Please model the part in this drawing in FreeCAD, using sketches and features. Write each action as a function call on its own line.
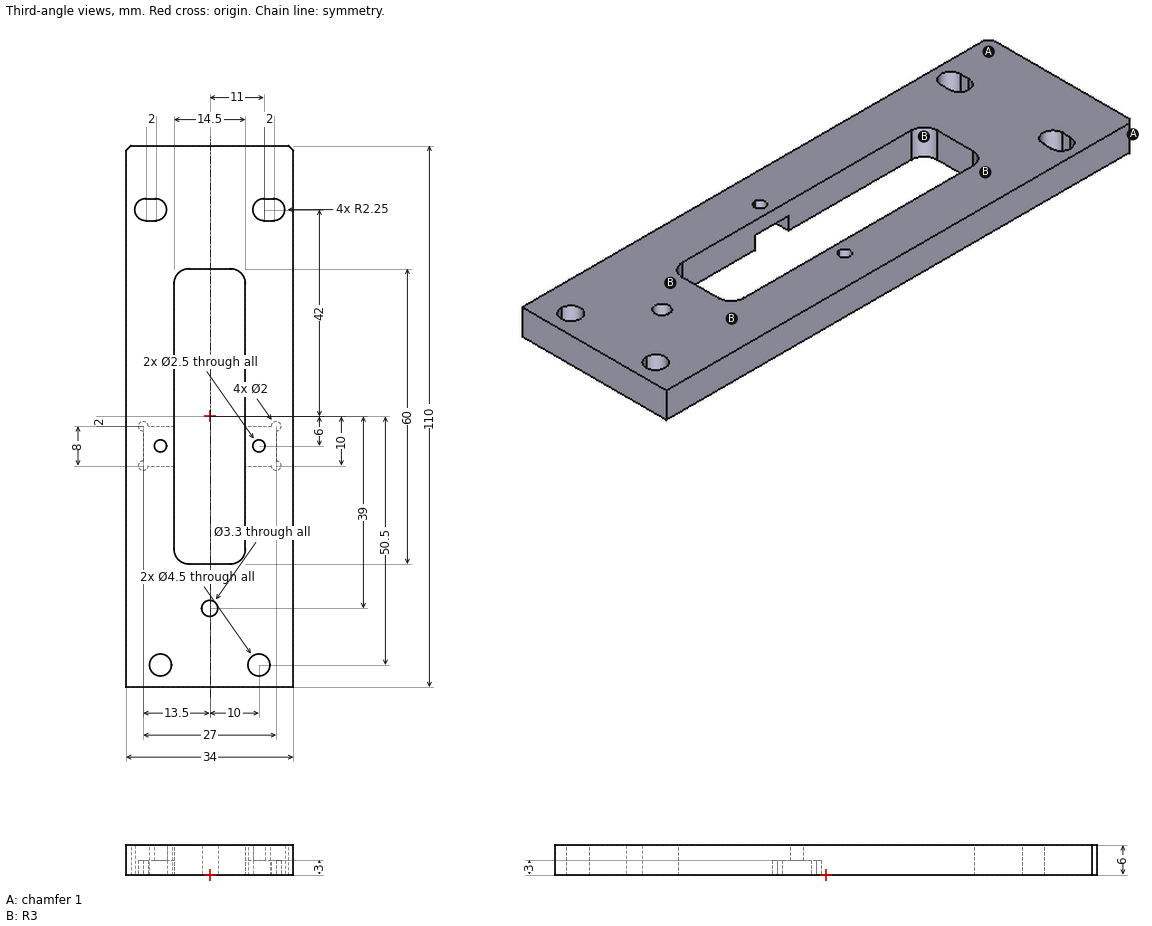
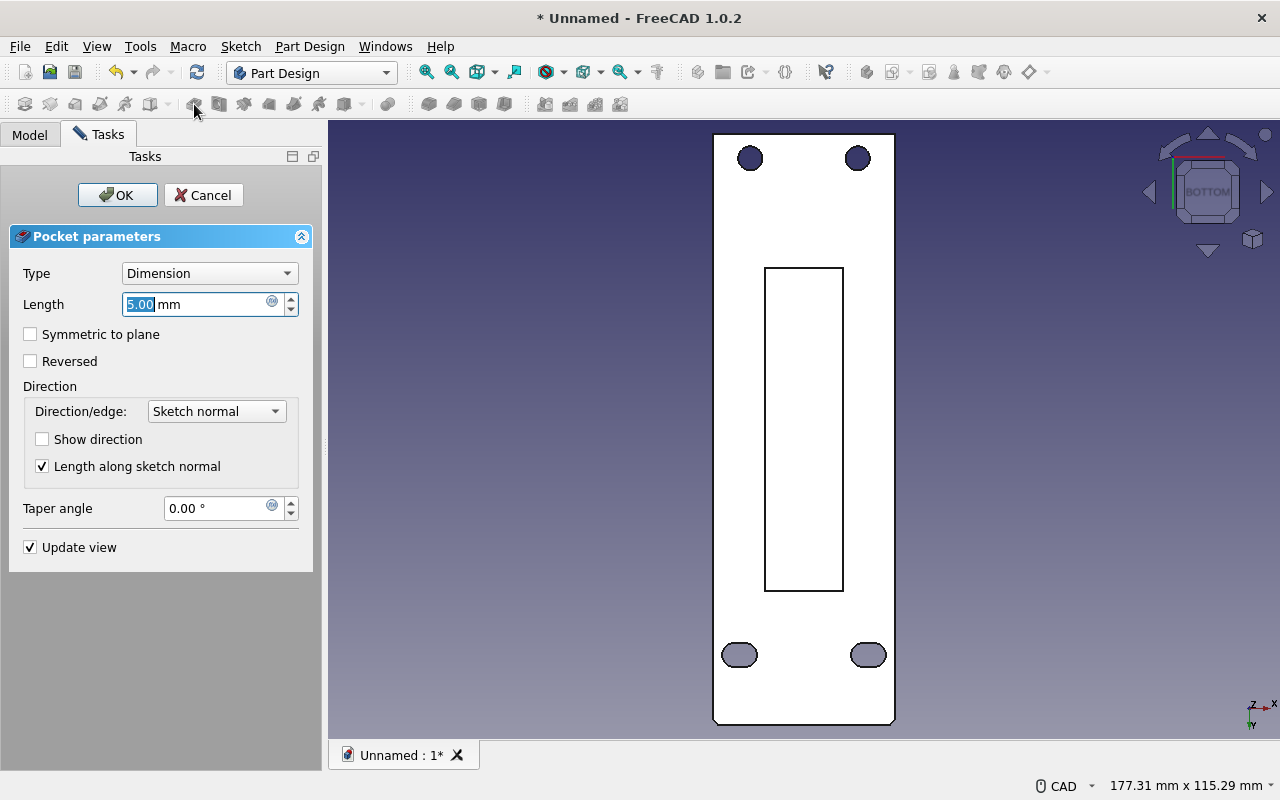
click(210, 274)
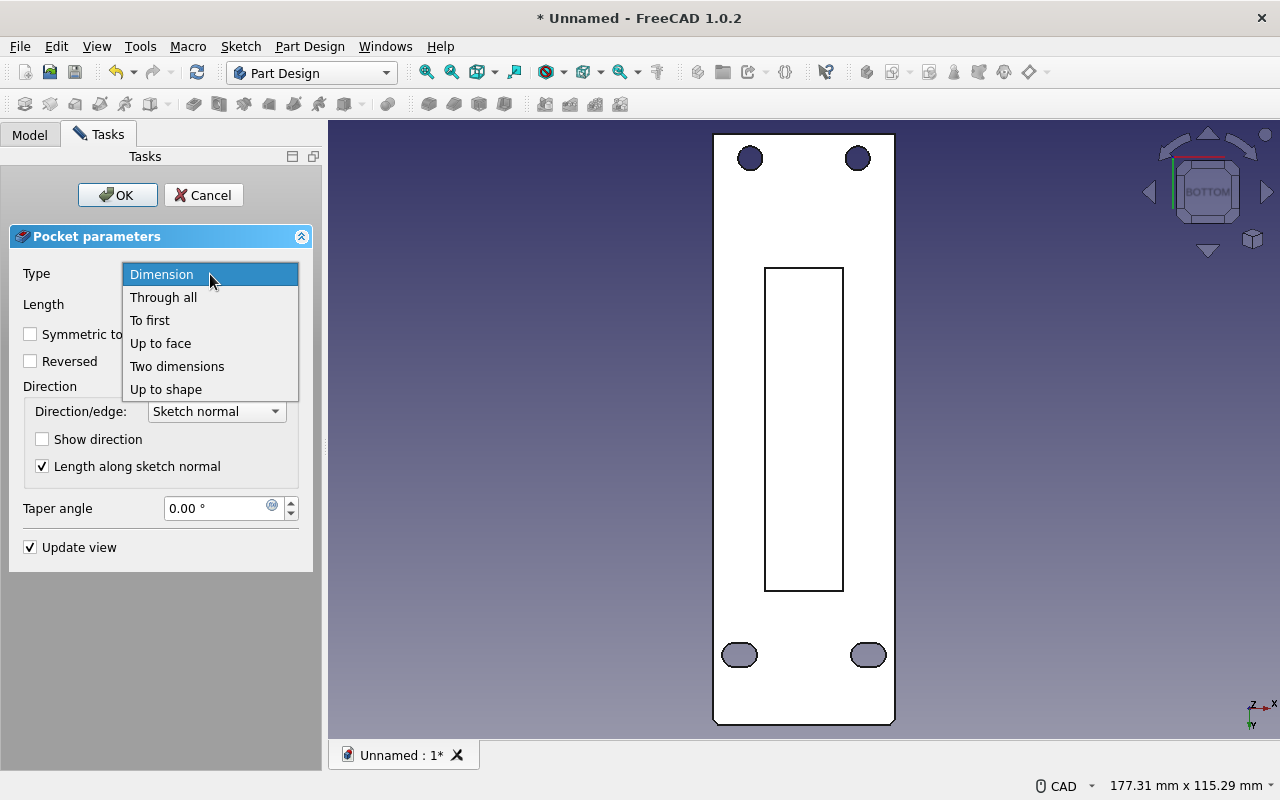
click(208, 298)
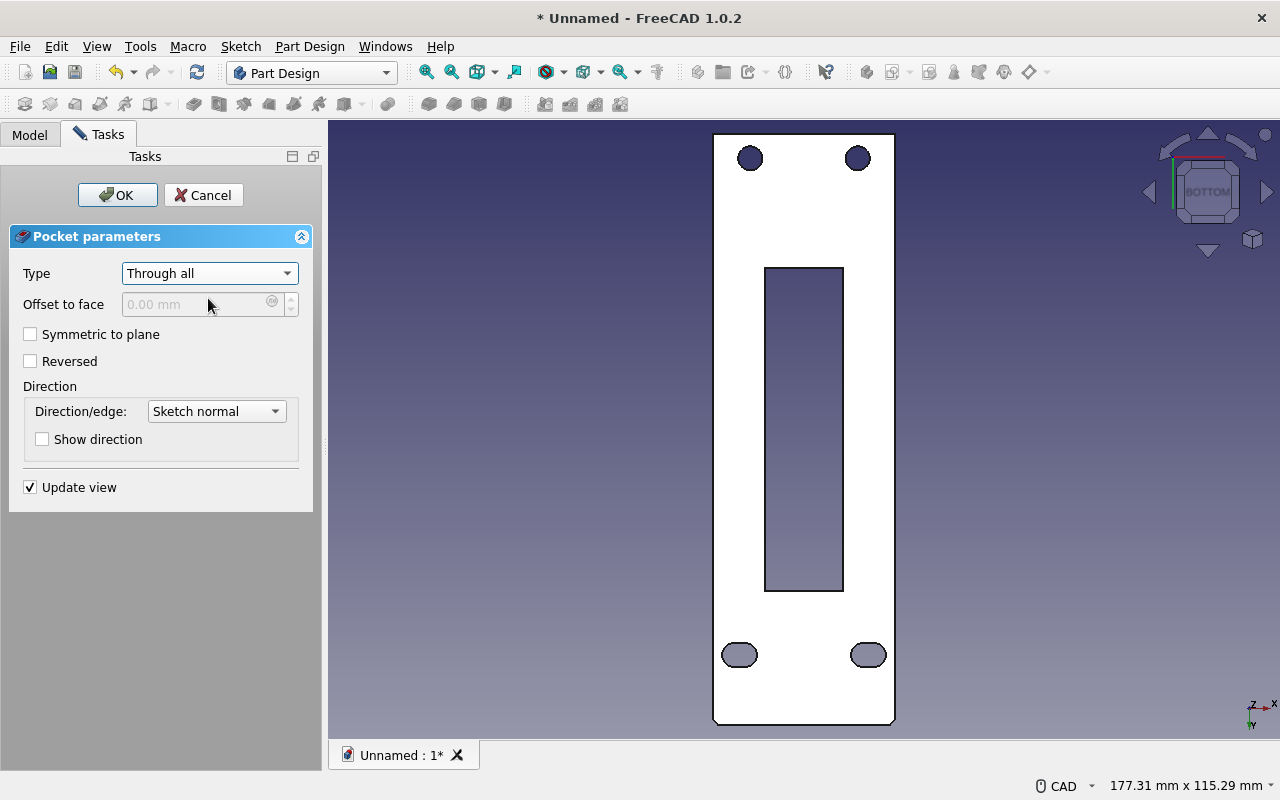
click(118, 195)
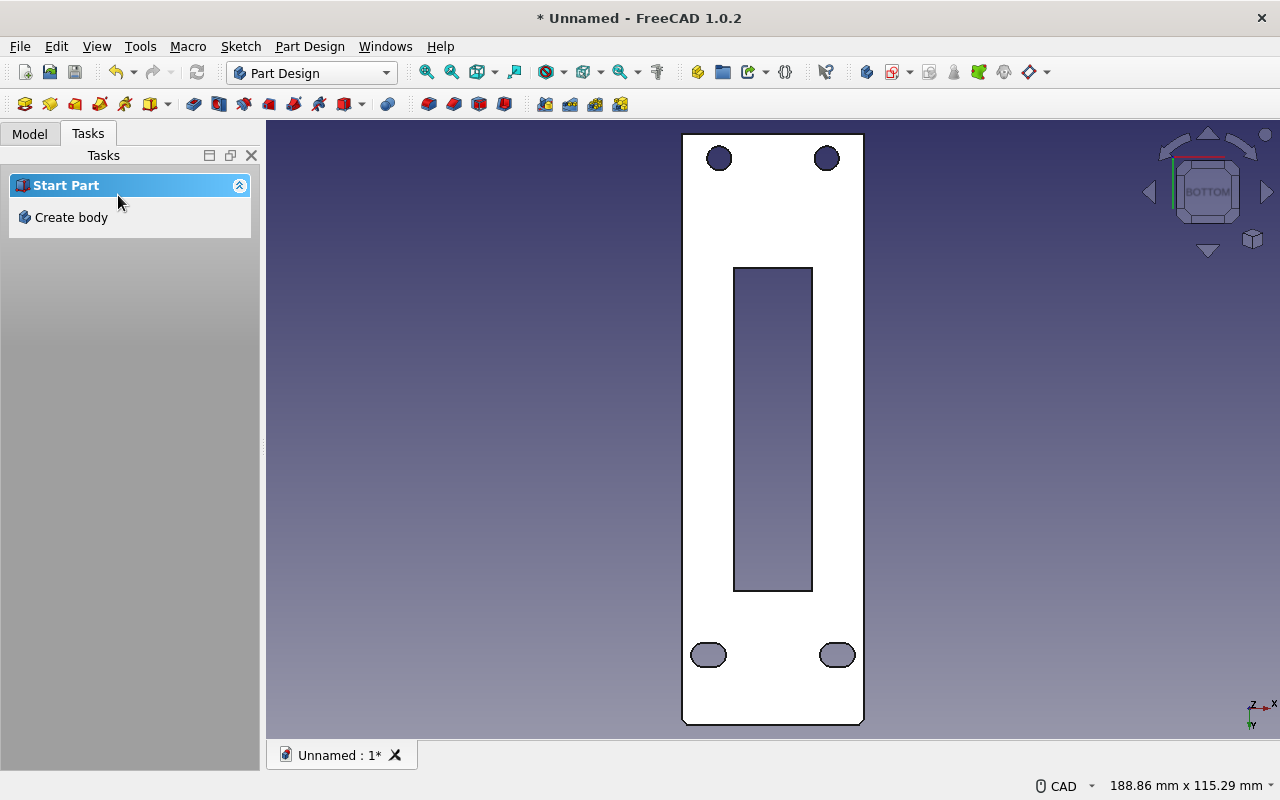
click(773, 682)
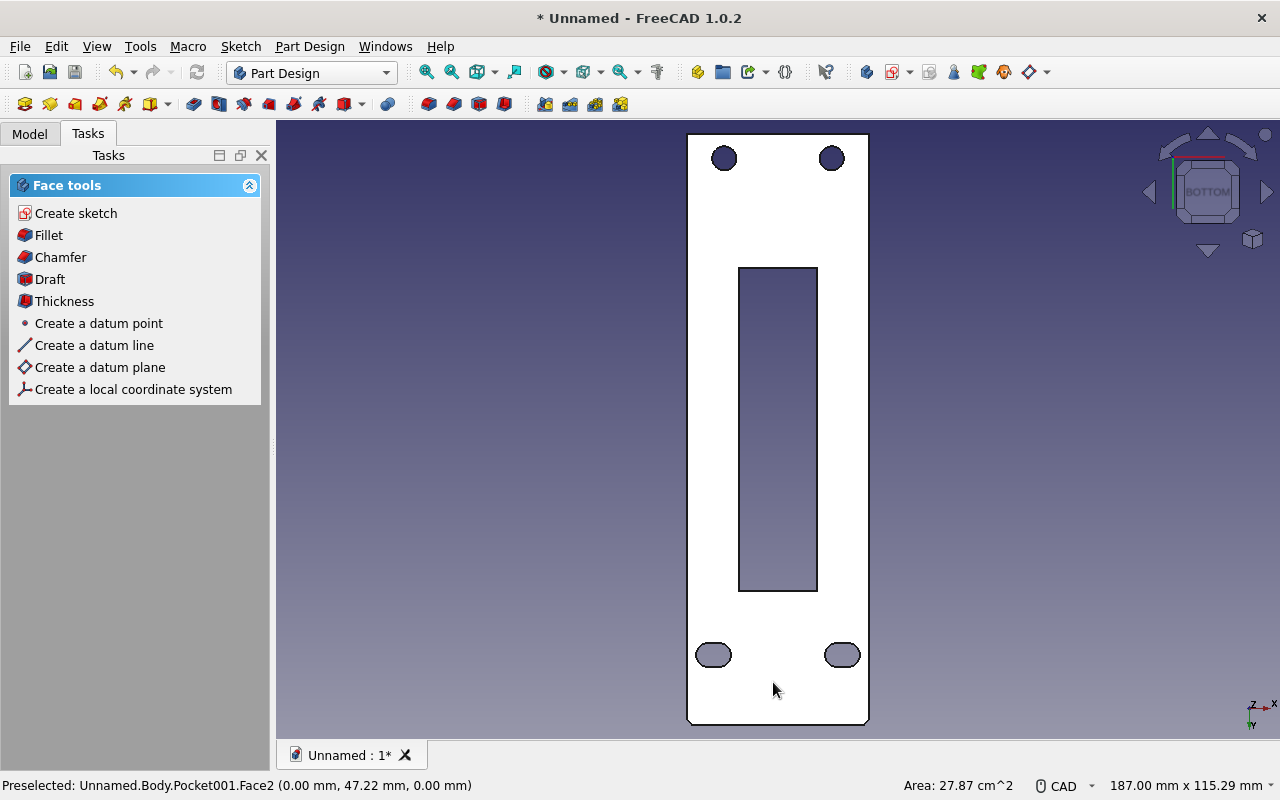
click(892, 72)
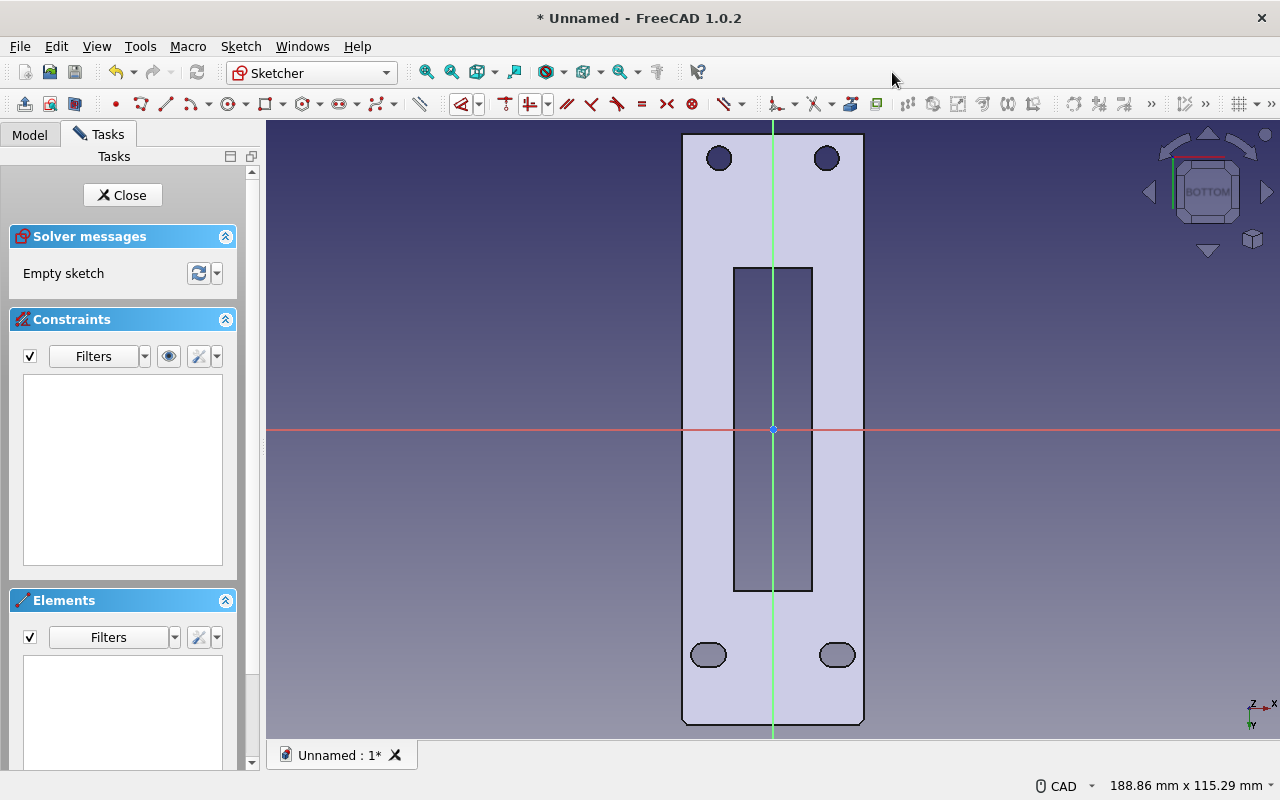
scroll(795, 394, up, 7)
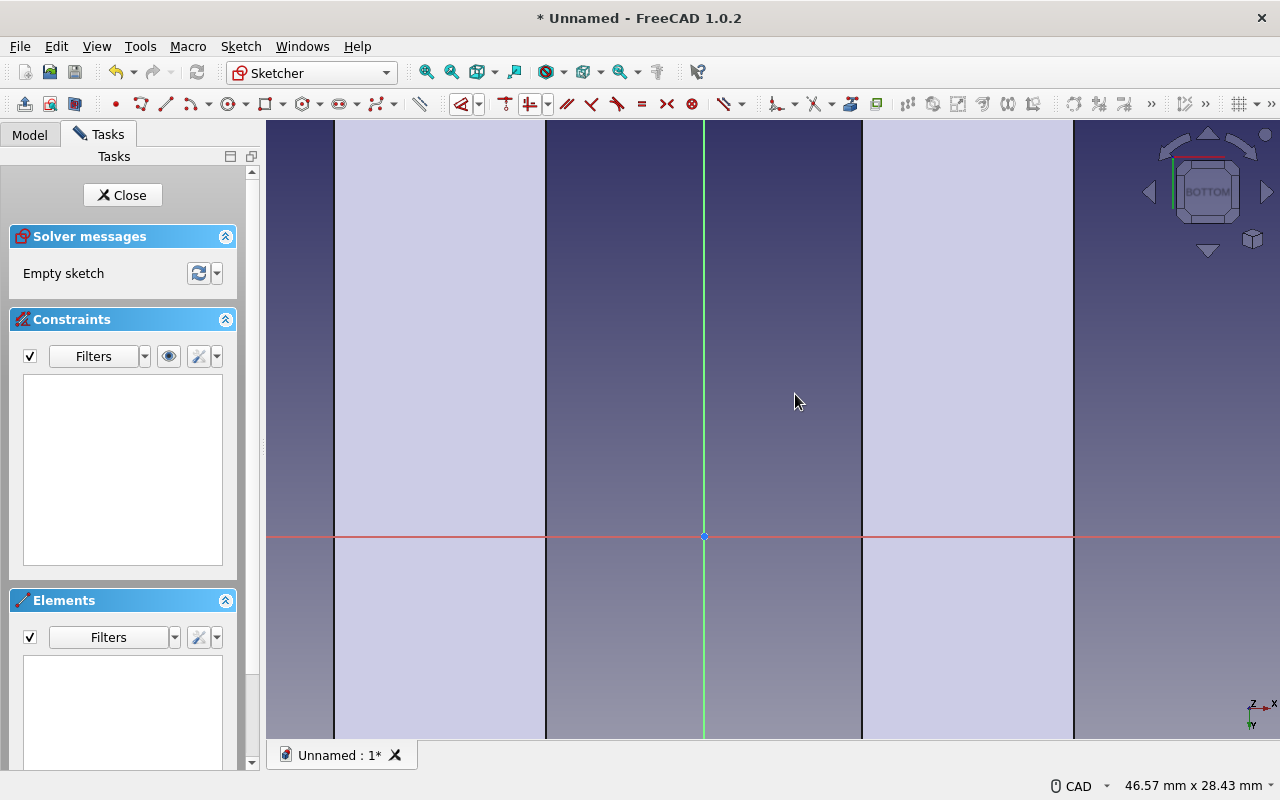
key(g)
key(r)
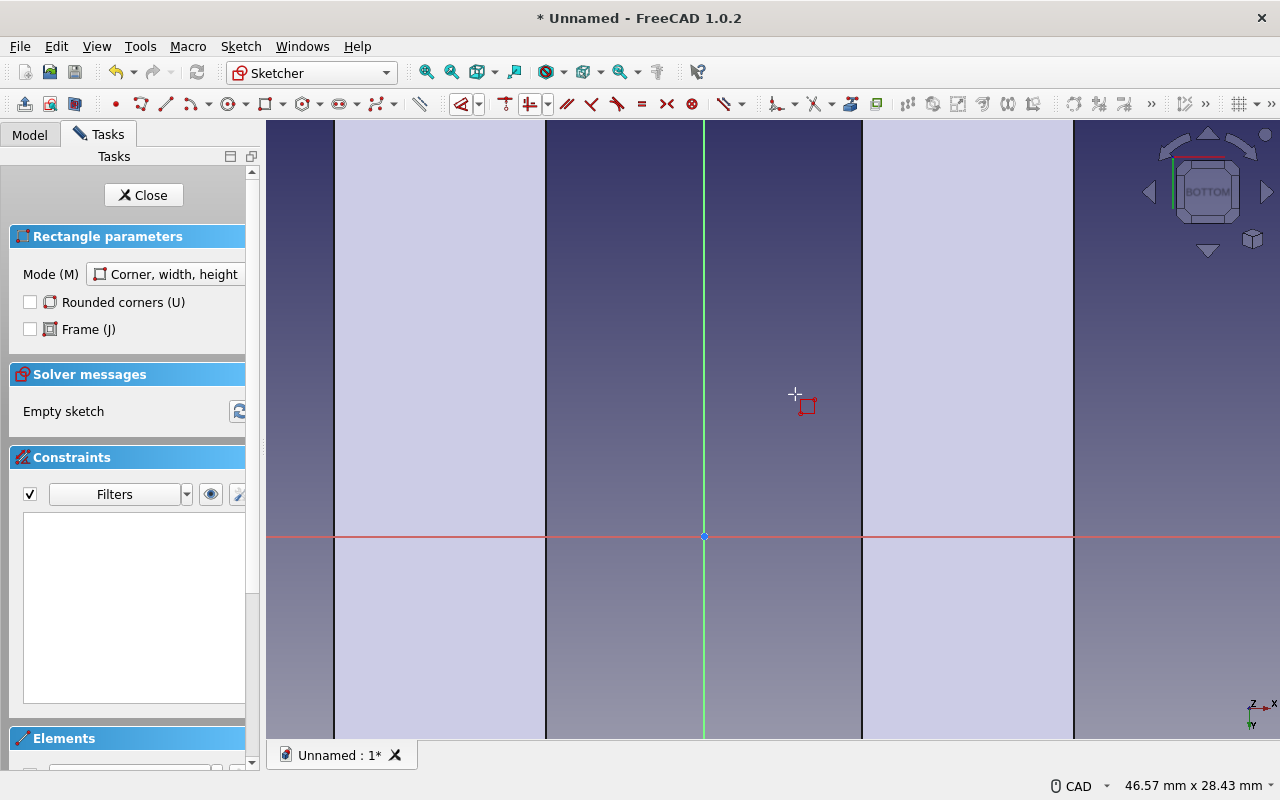
click(410, 319)
click(998, 493)
key(Escape)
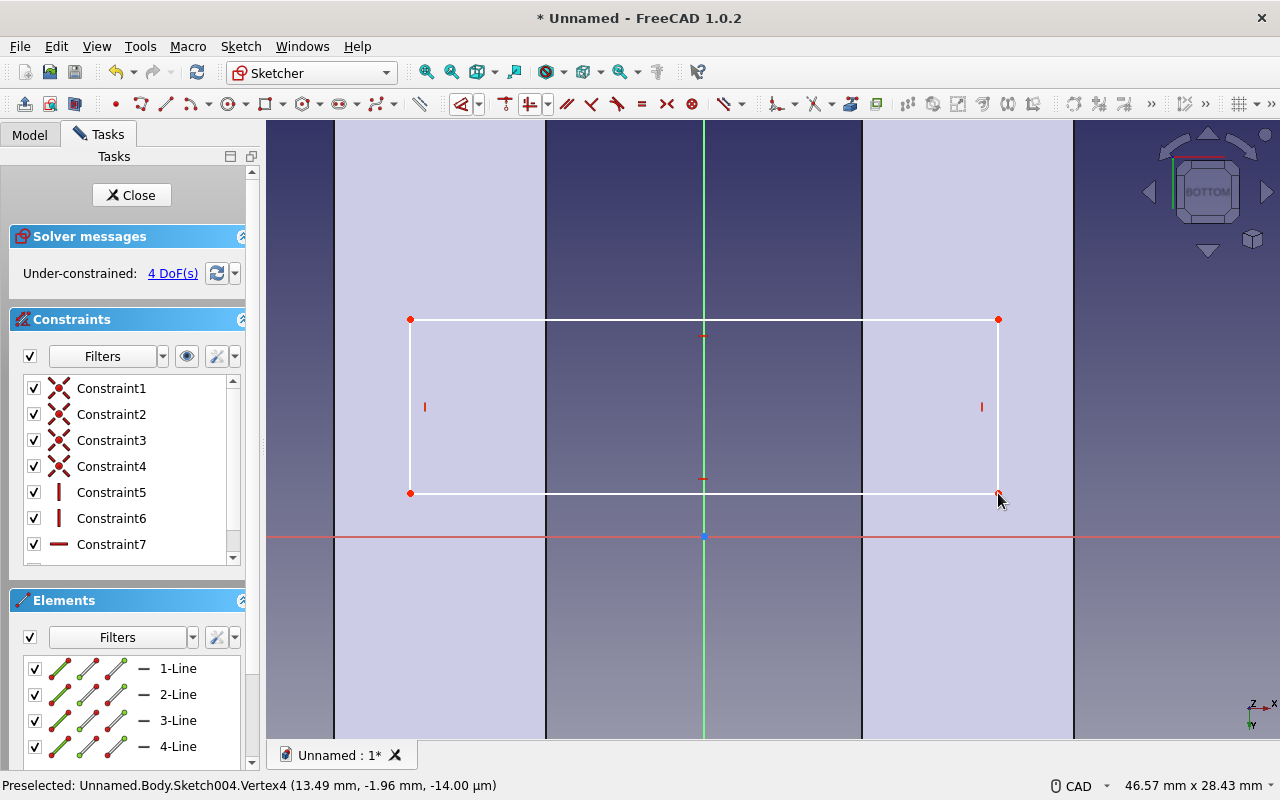
click(410, 372)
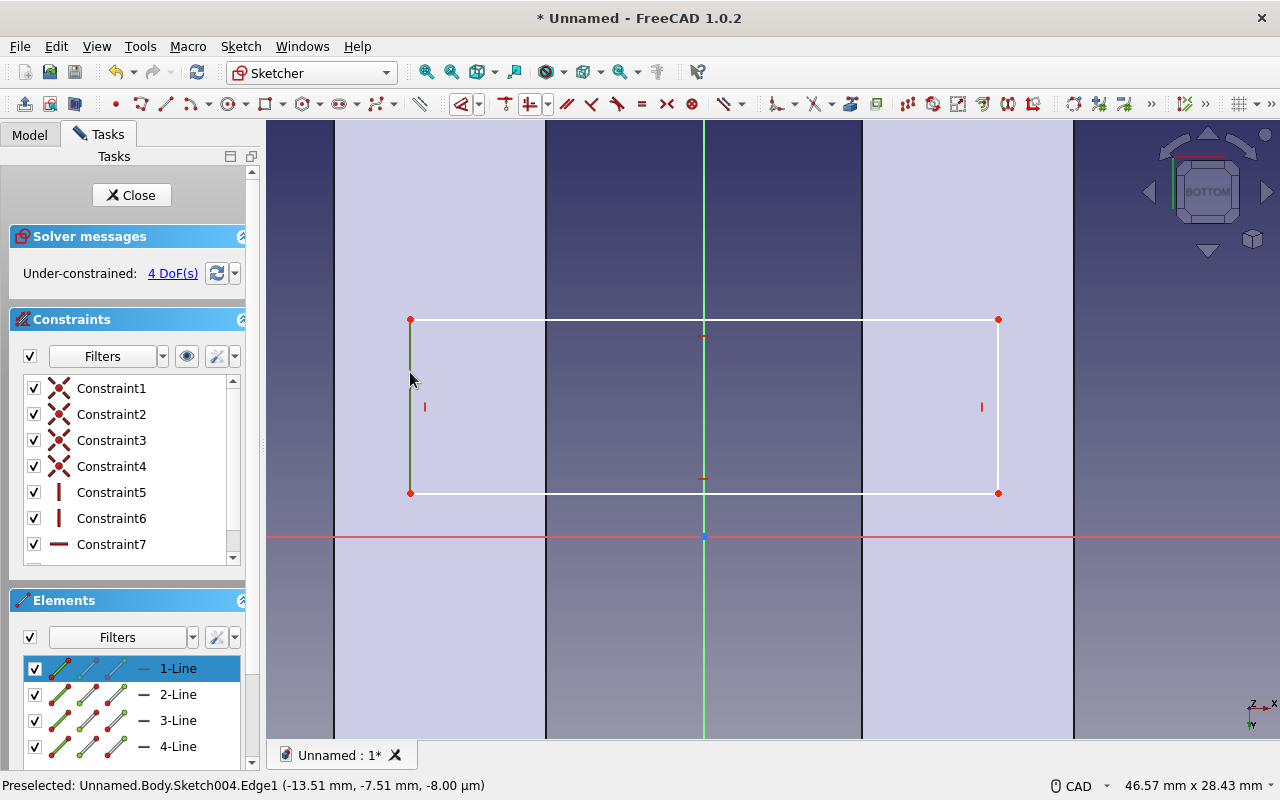
key(i)